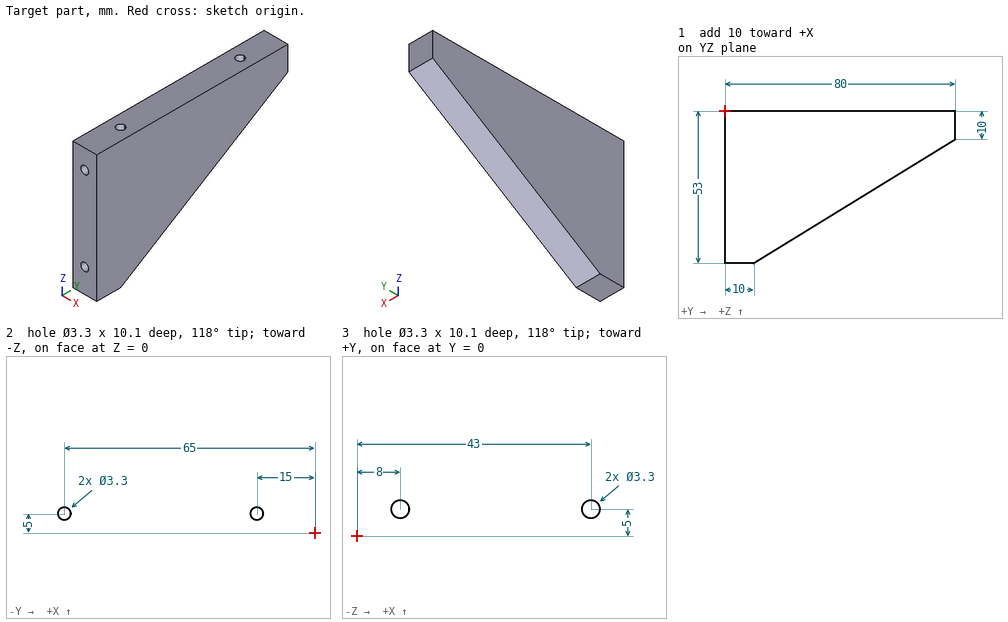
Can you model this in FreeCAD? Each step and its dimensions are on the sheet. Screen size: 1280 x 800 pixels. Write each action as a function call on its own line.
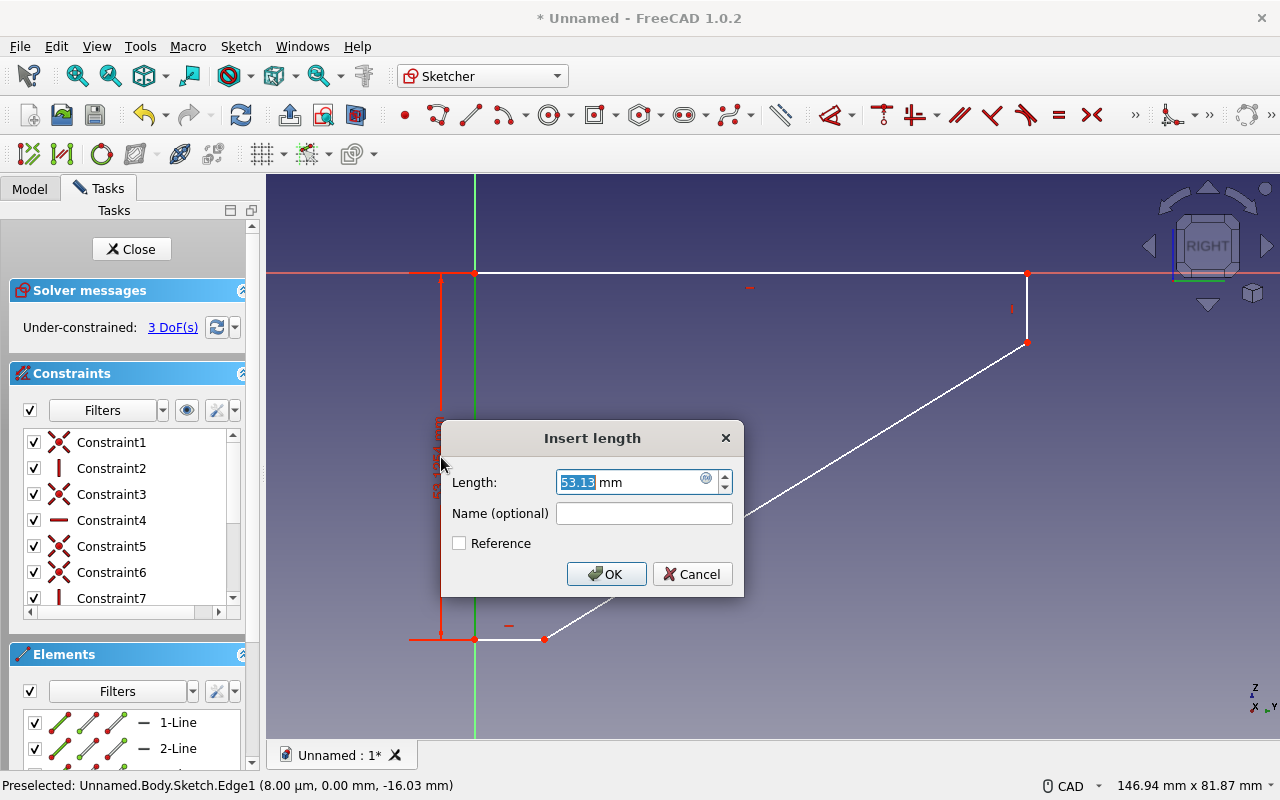
text(53)
key(Return)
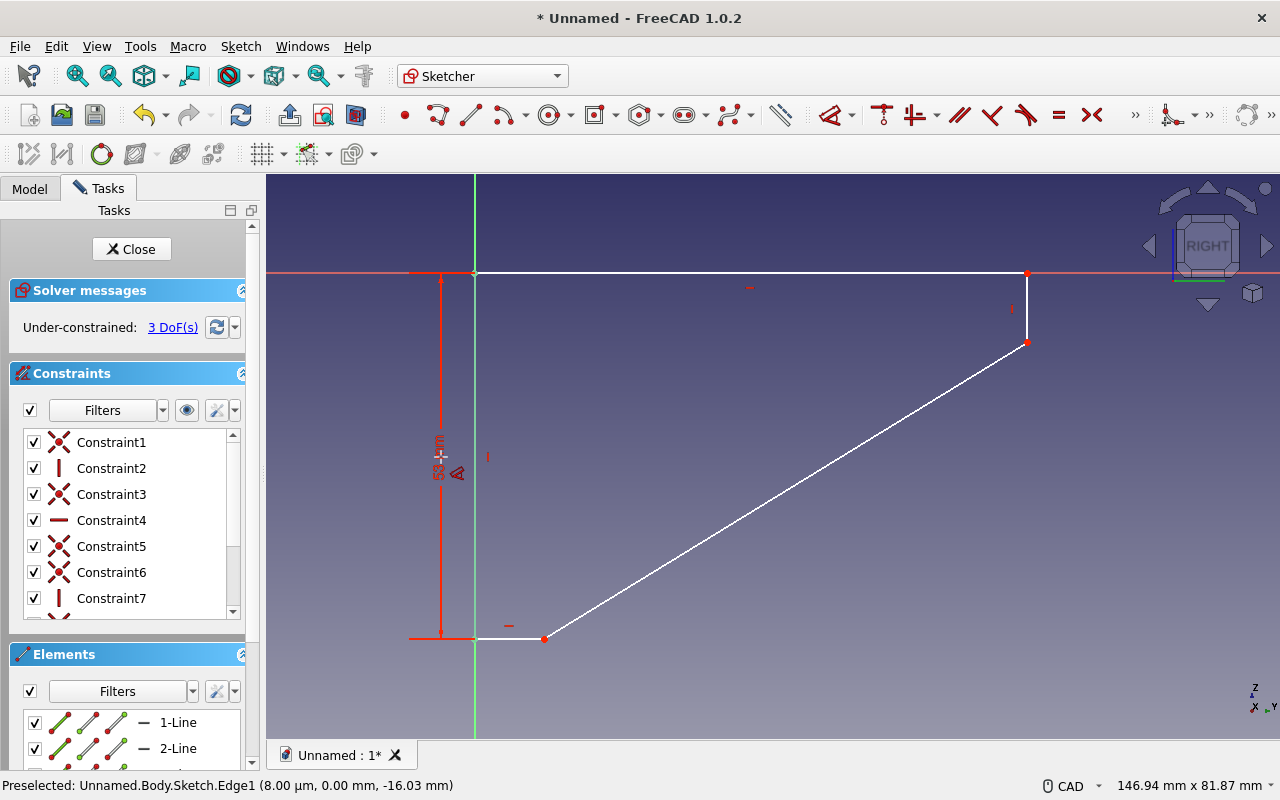
click(496, 639)
click(509, 673)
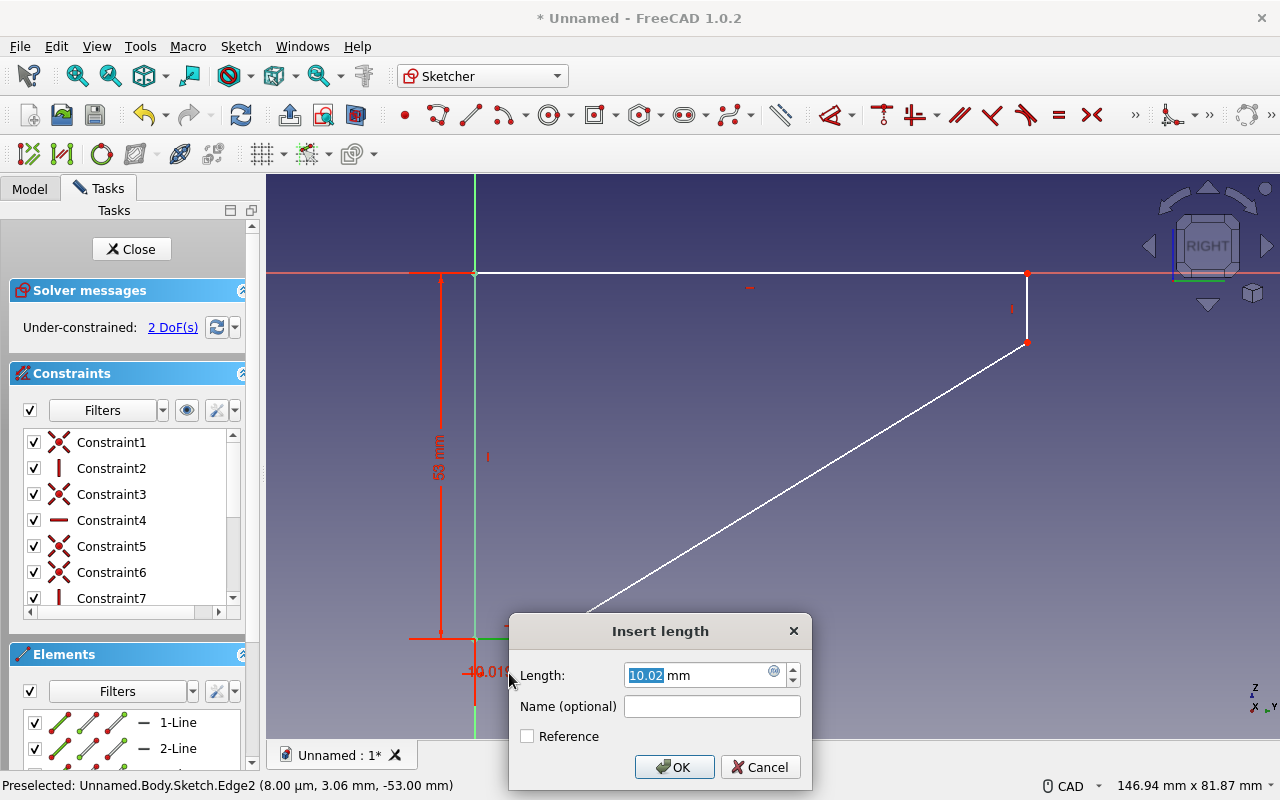
text(10)
key(Return)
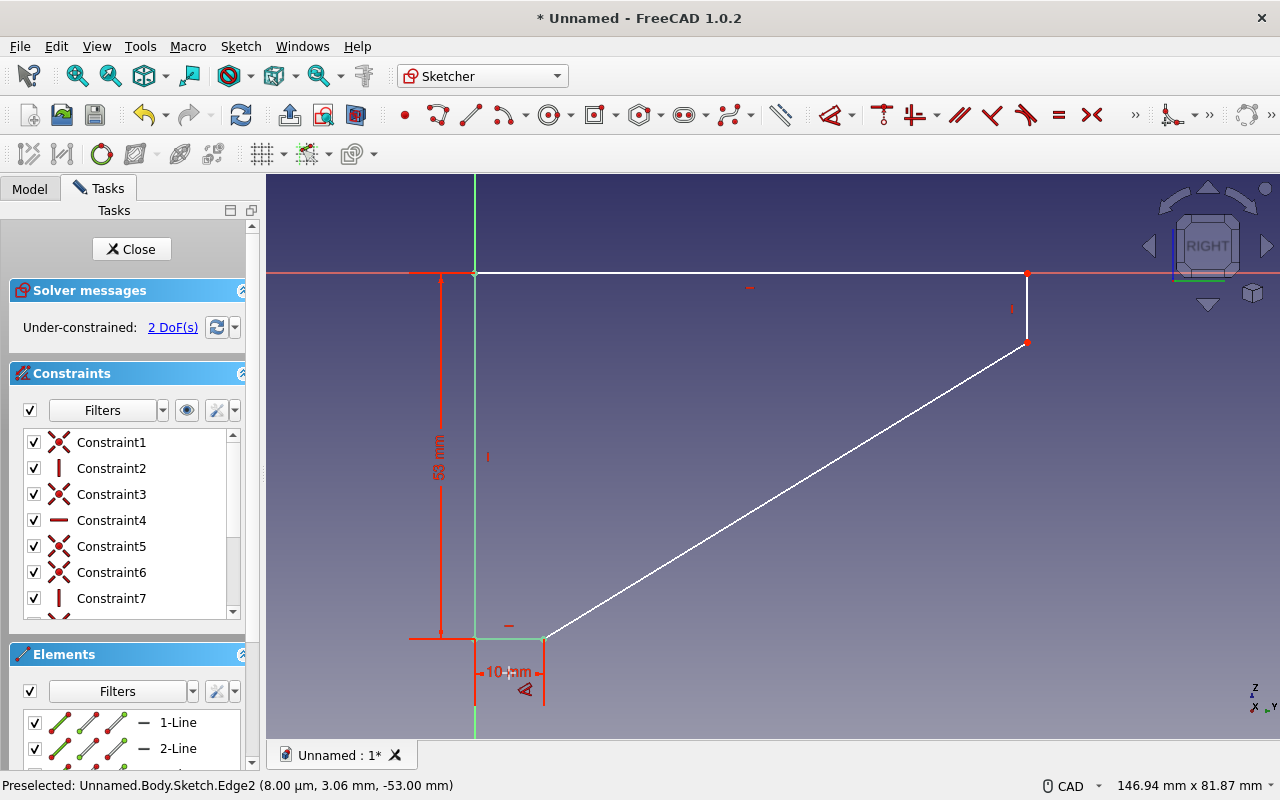
click(1027, 322)
click(1061, 308)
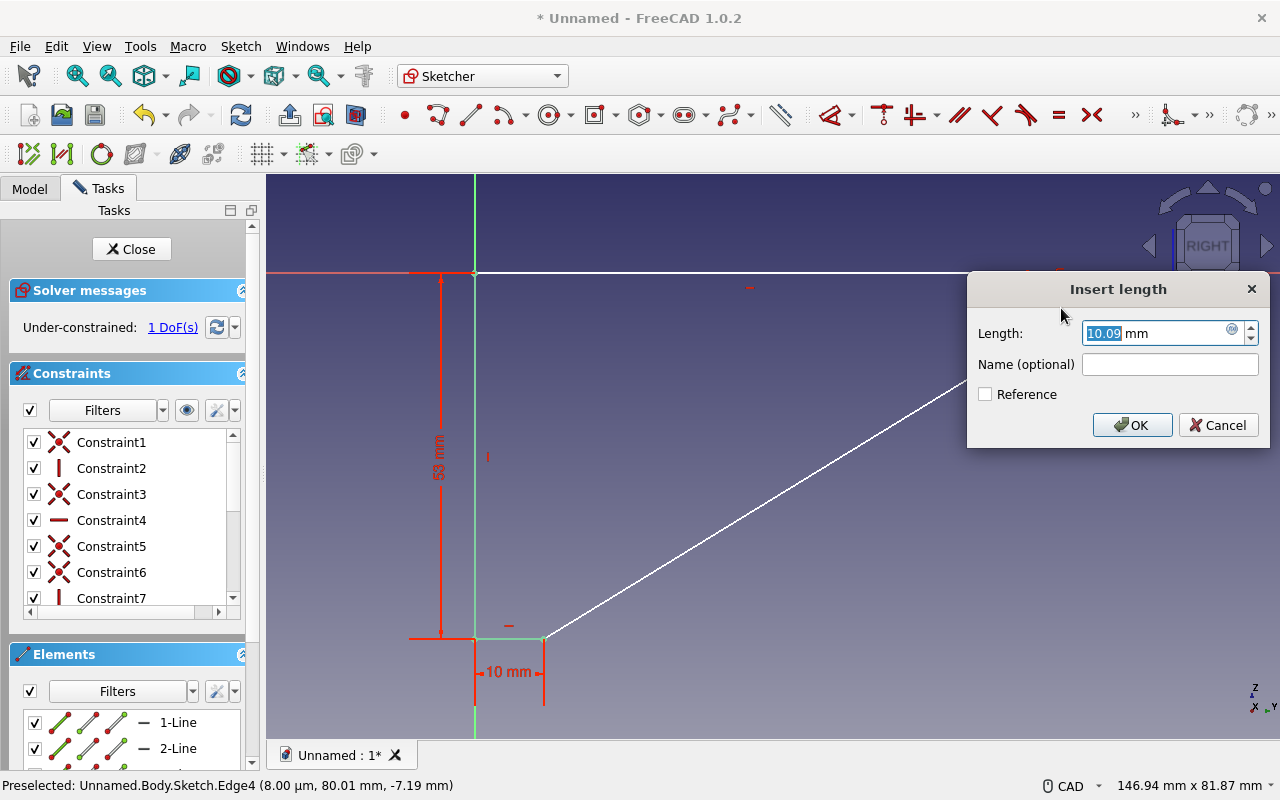
text(10)
key(Return)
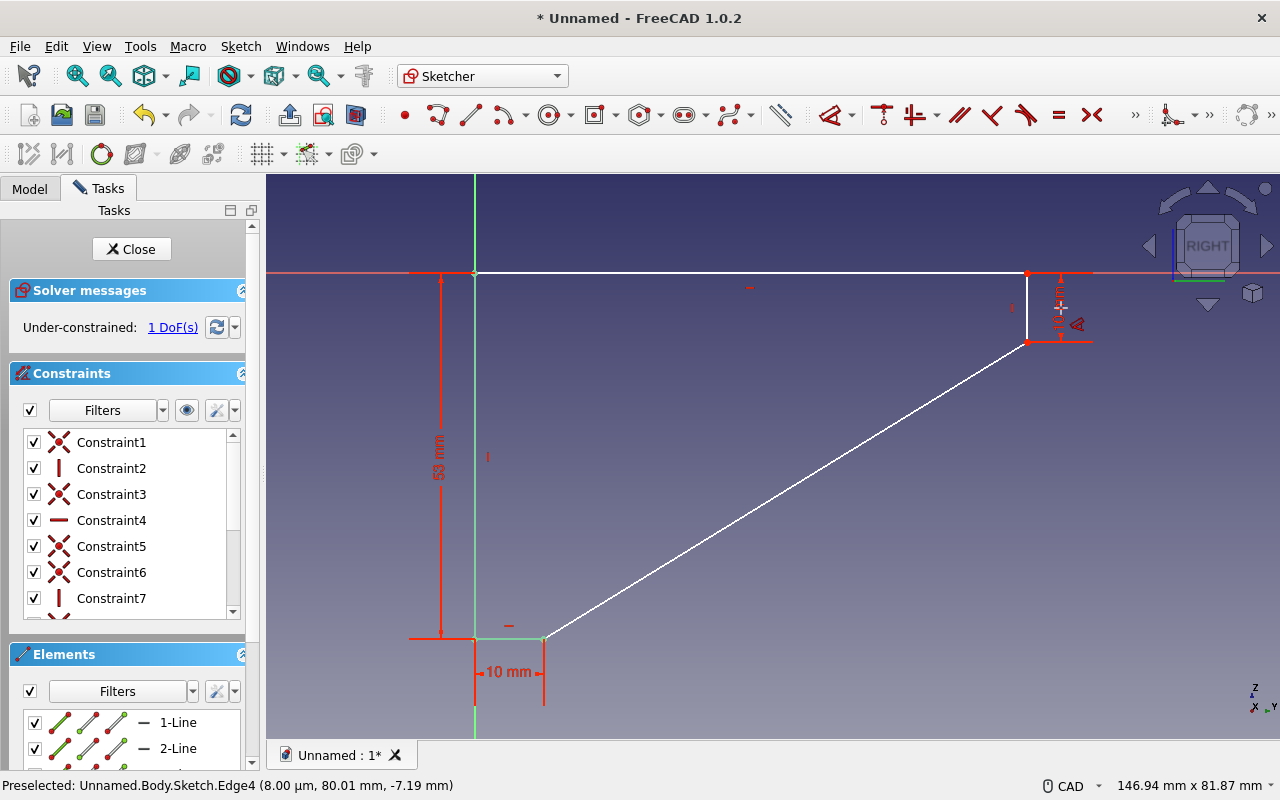
click(861, 273)
click(751, 239)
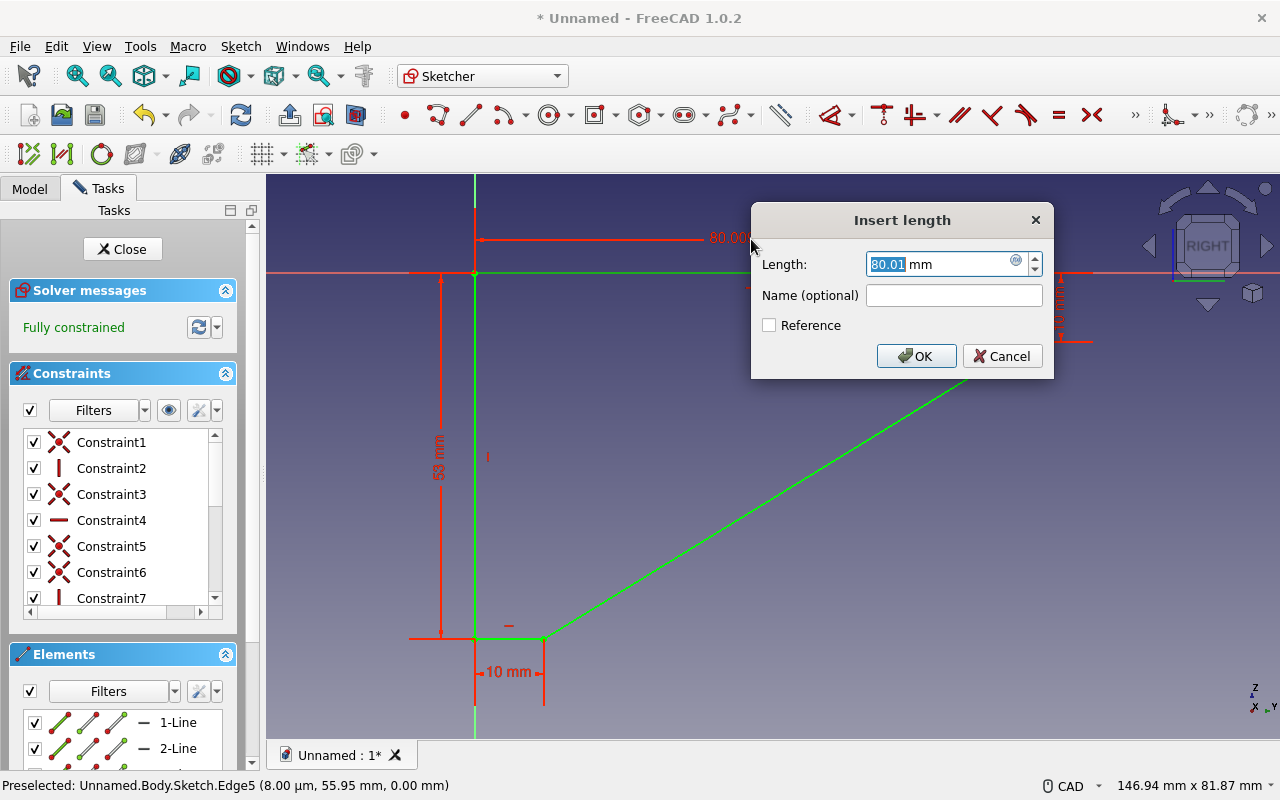
text(80)
key(Return)
key(Escape)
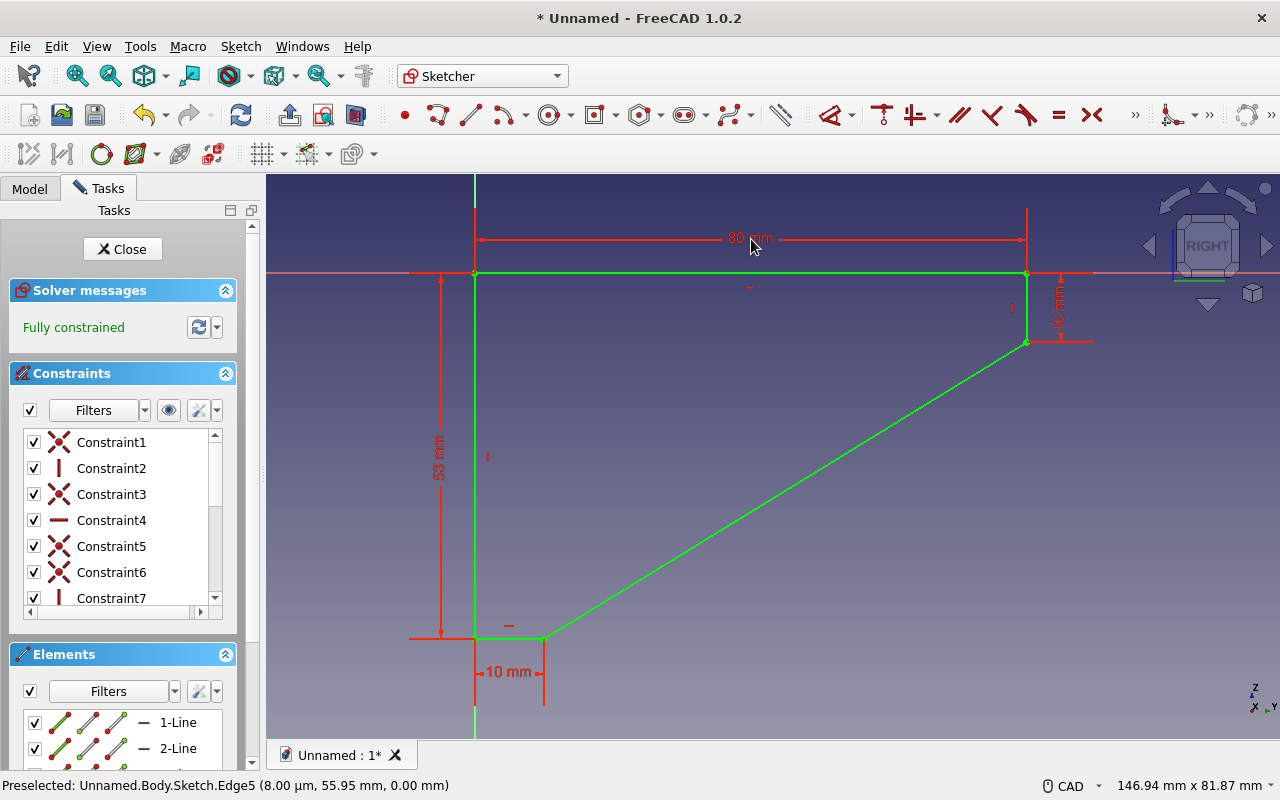
click(123, 249)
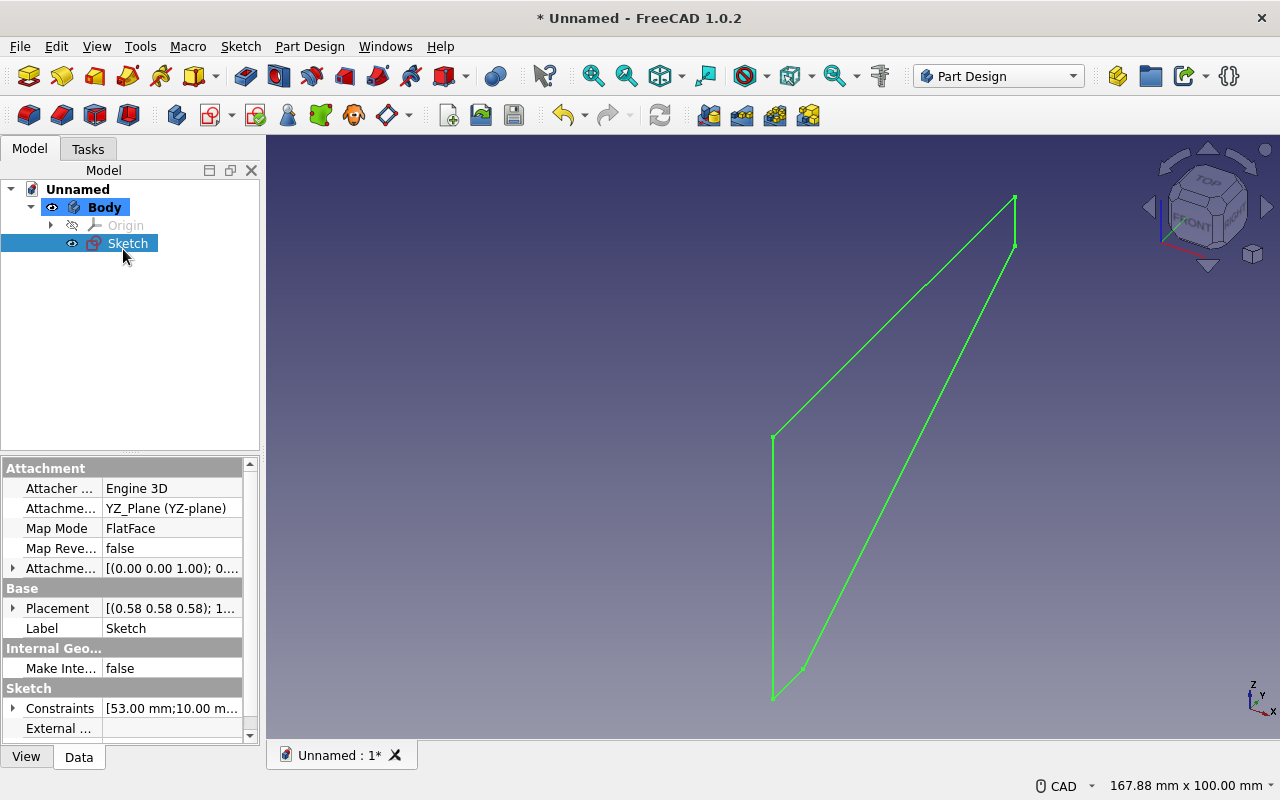
click(29, 76)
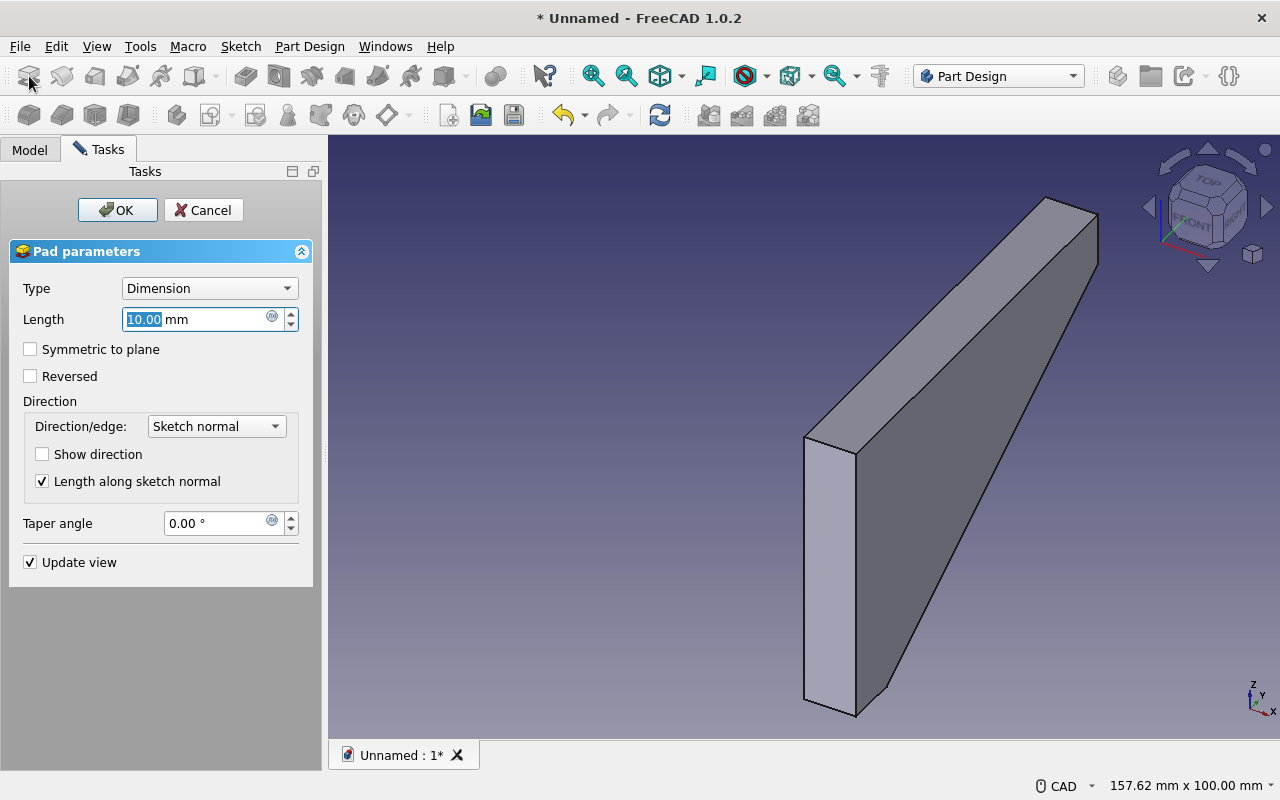
text(10)
key(Tab)